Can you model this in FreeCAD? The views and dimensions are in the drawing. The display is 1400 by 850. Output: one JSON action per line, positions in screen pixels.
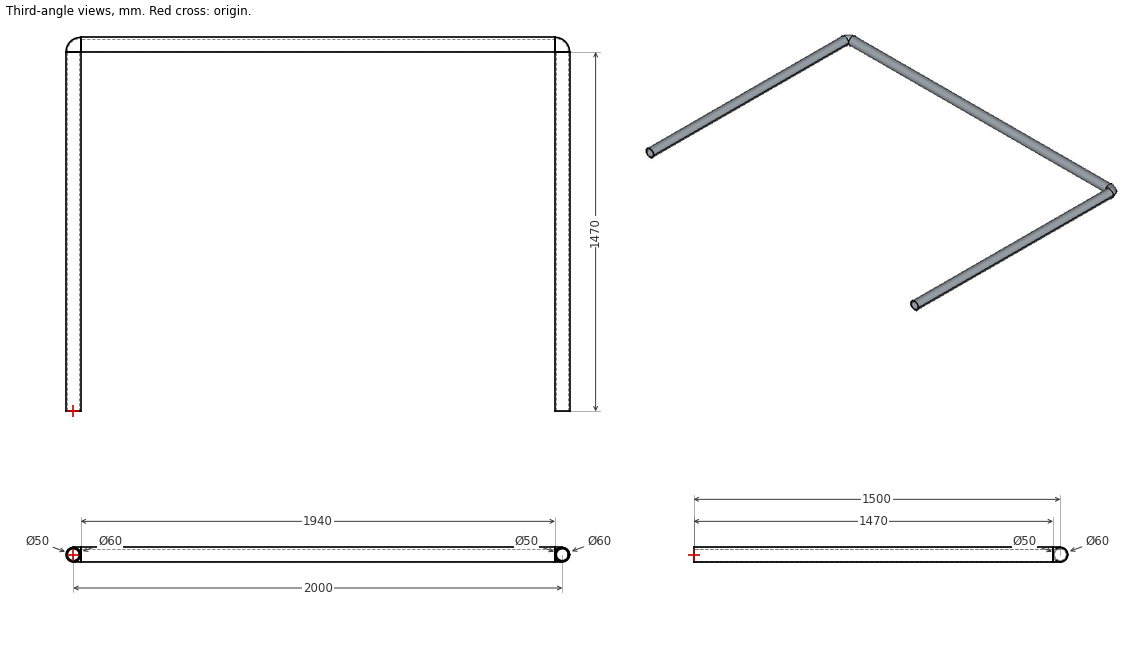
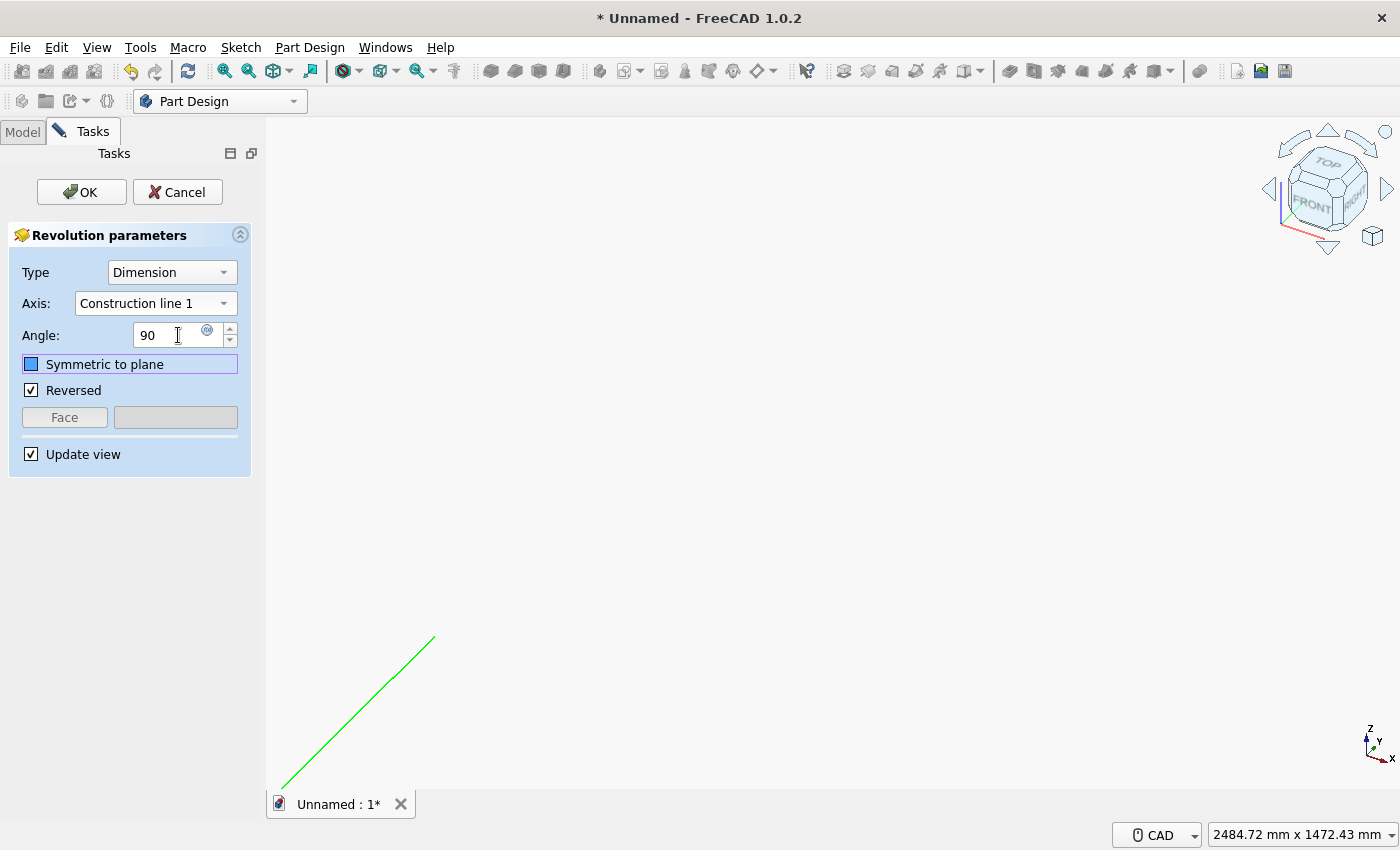
{"action": "left_click", "coordinate": [30, 390]}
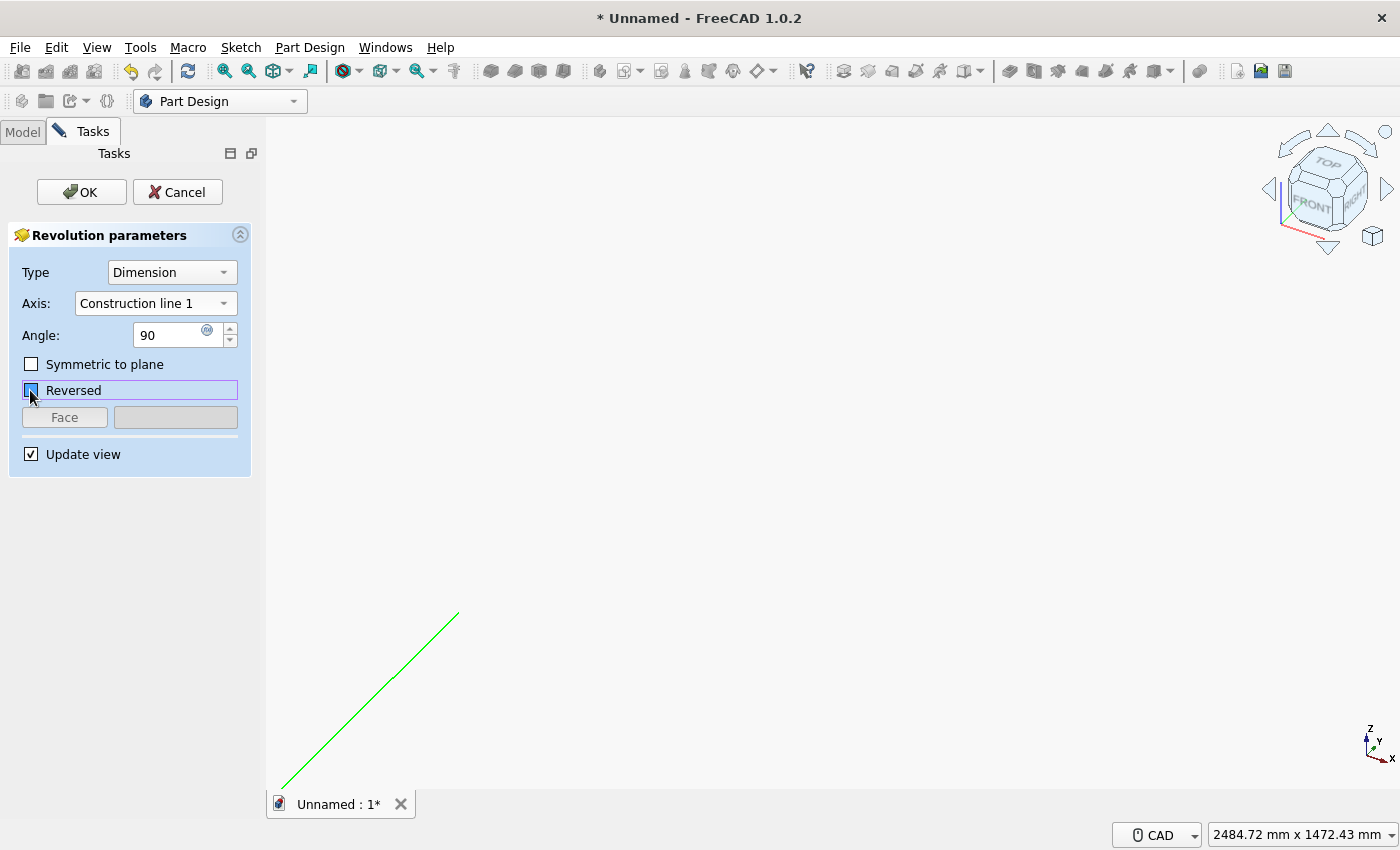
{"action": "left_click", "coordinate": [82, 192]}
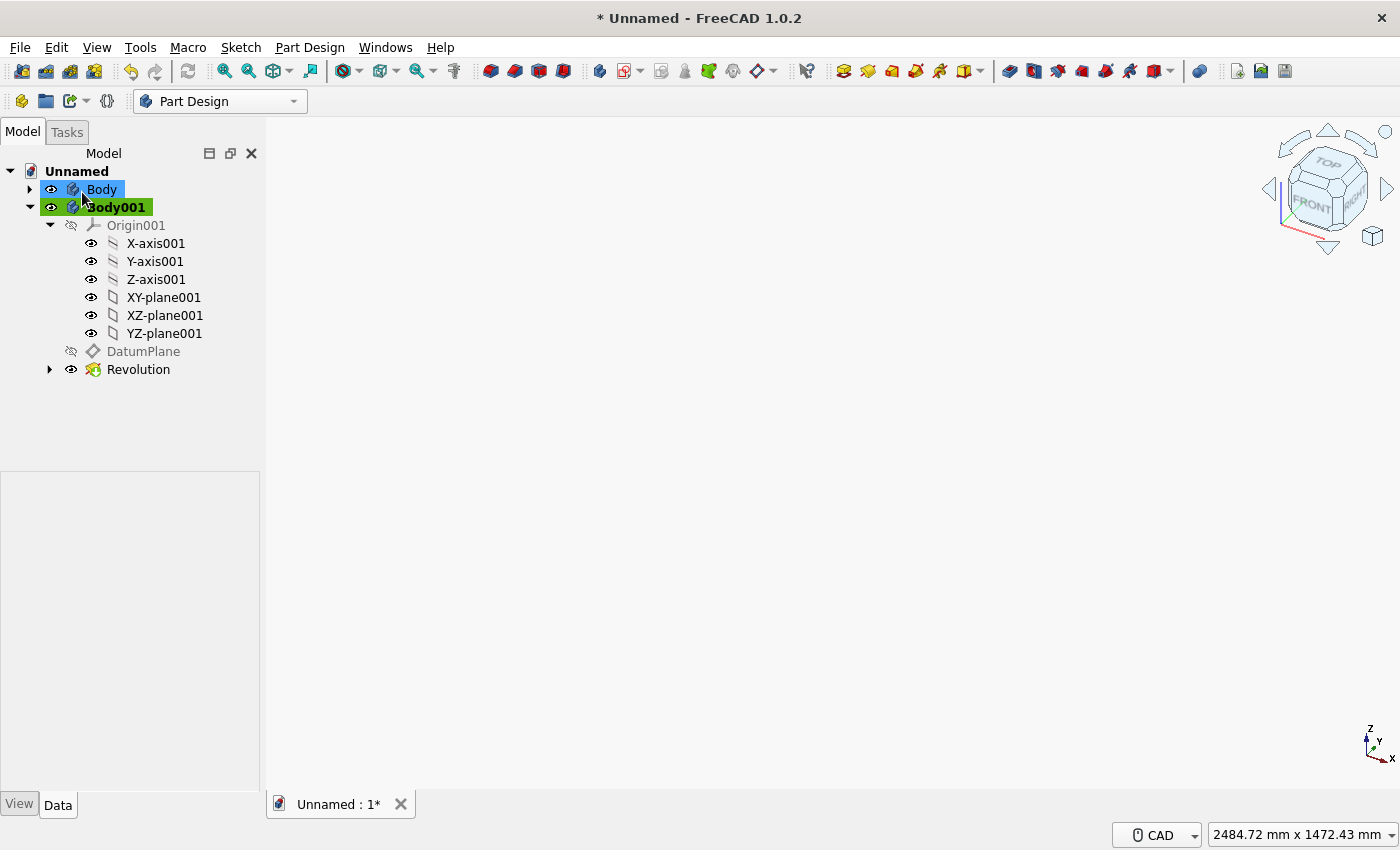
{"action": "left_click", "coordinate": [226, 72]}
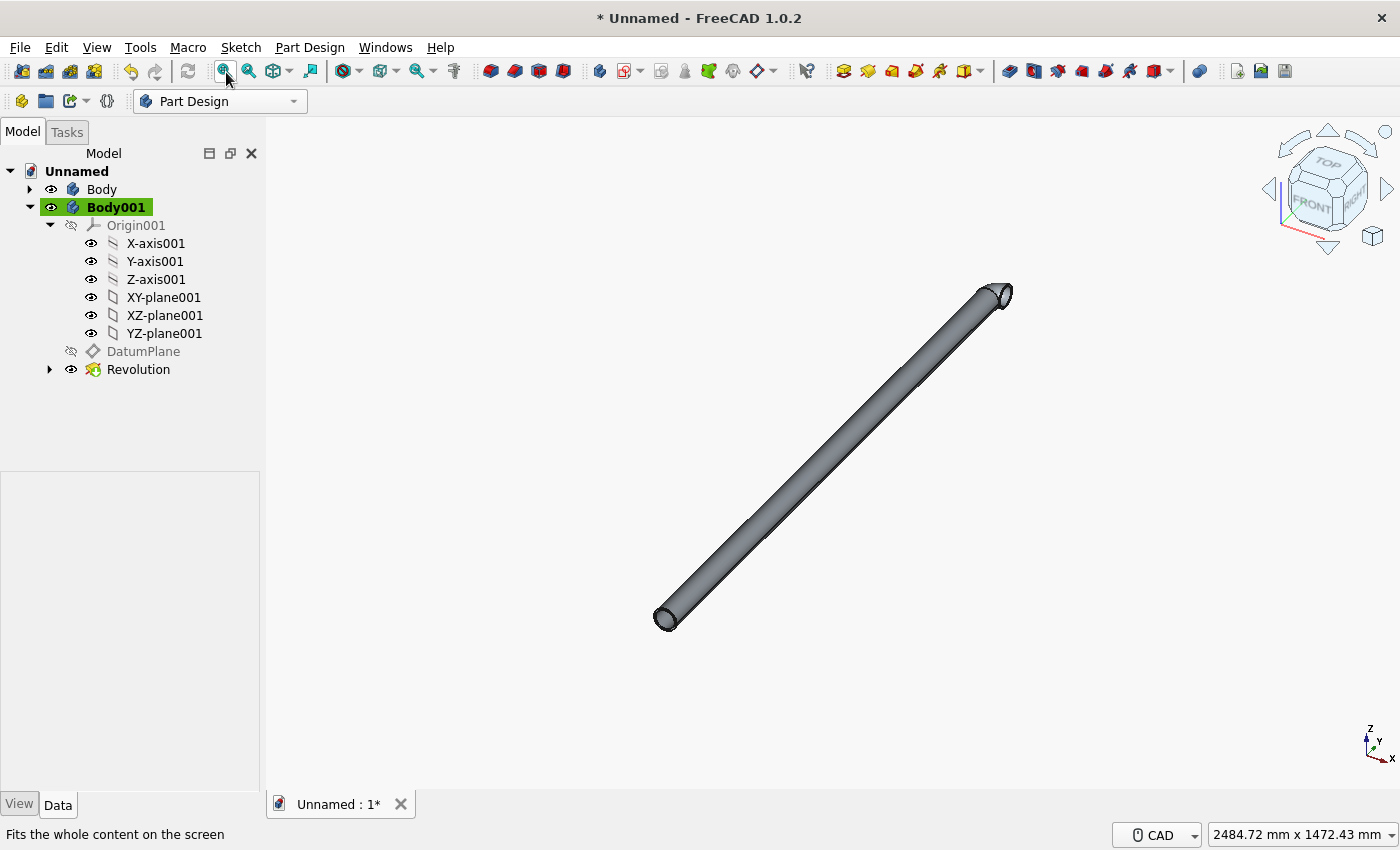
{"action": "left_click", "coordinate": [600, 72]}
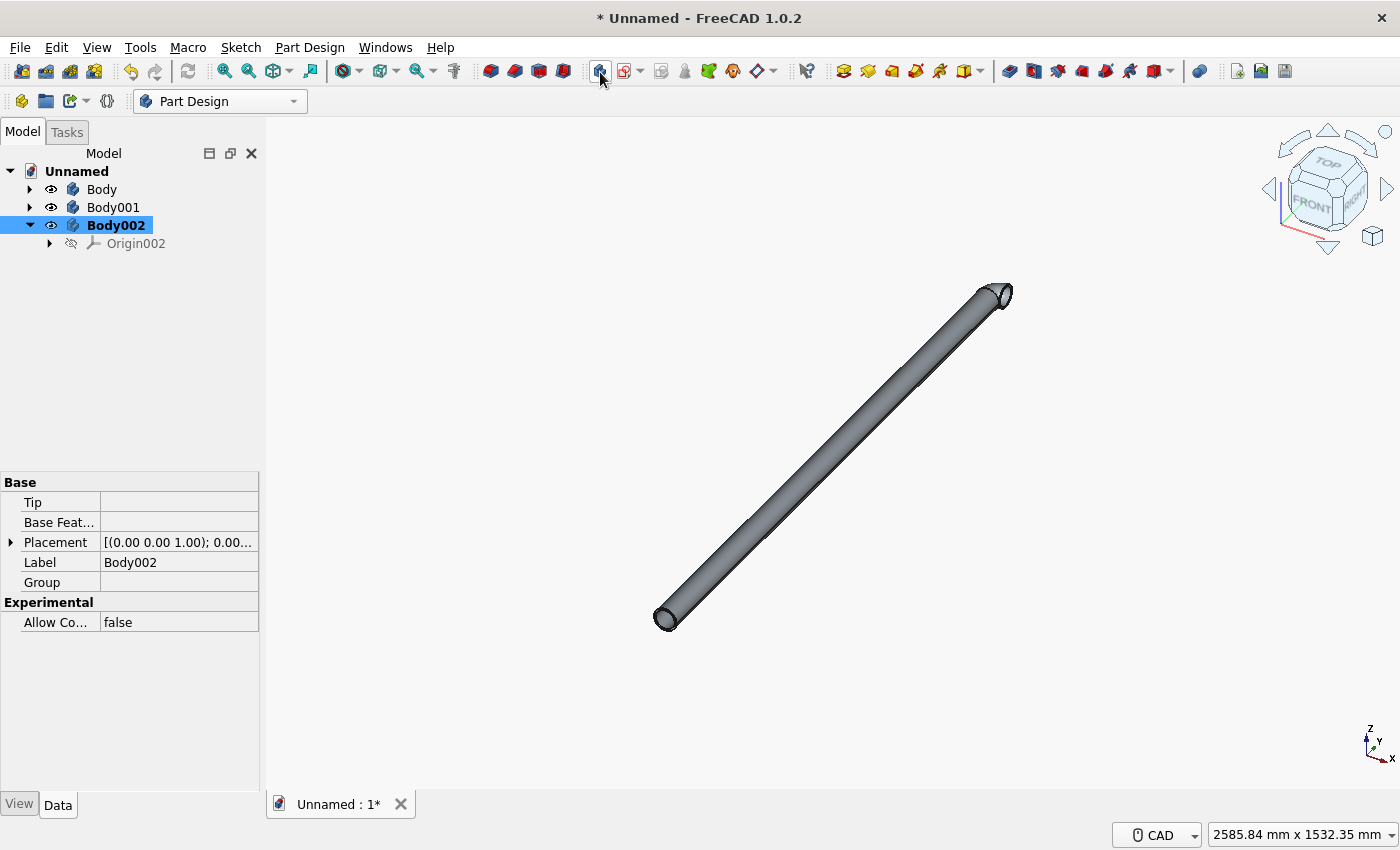
{"action": "left_click", "coordinate": [50, 243]}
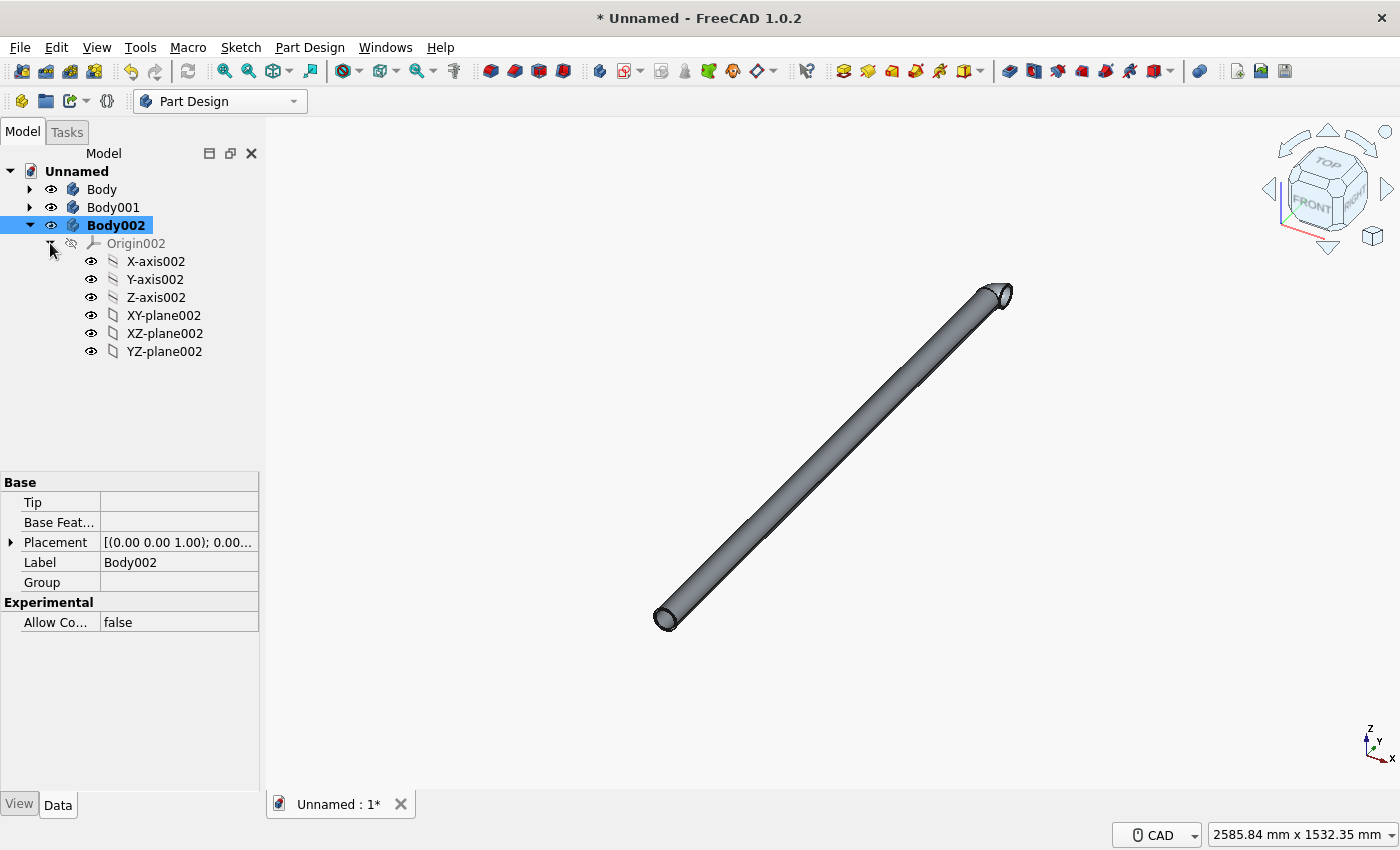
{"action": "left_click", "coordinate": [136, 351]}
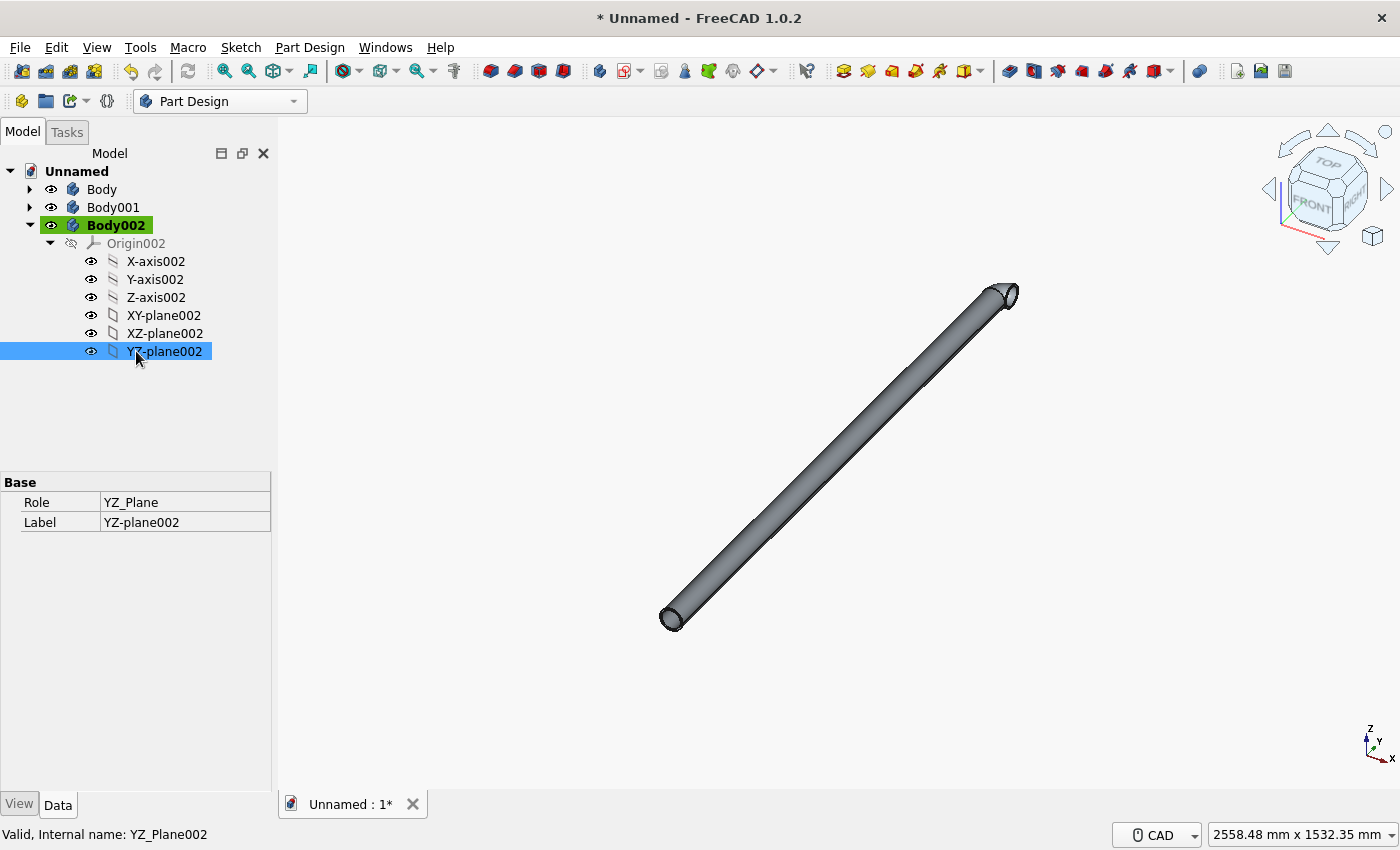
{"action": "left_click", "coordinate": [758, 72]}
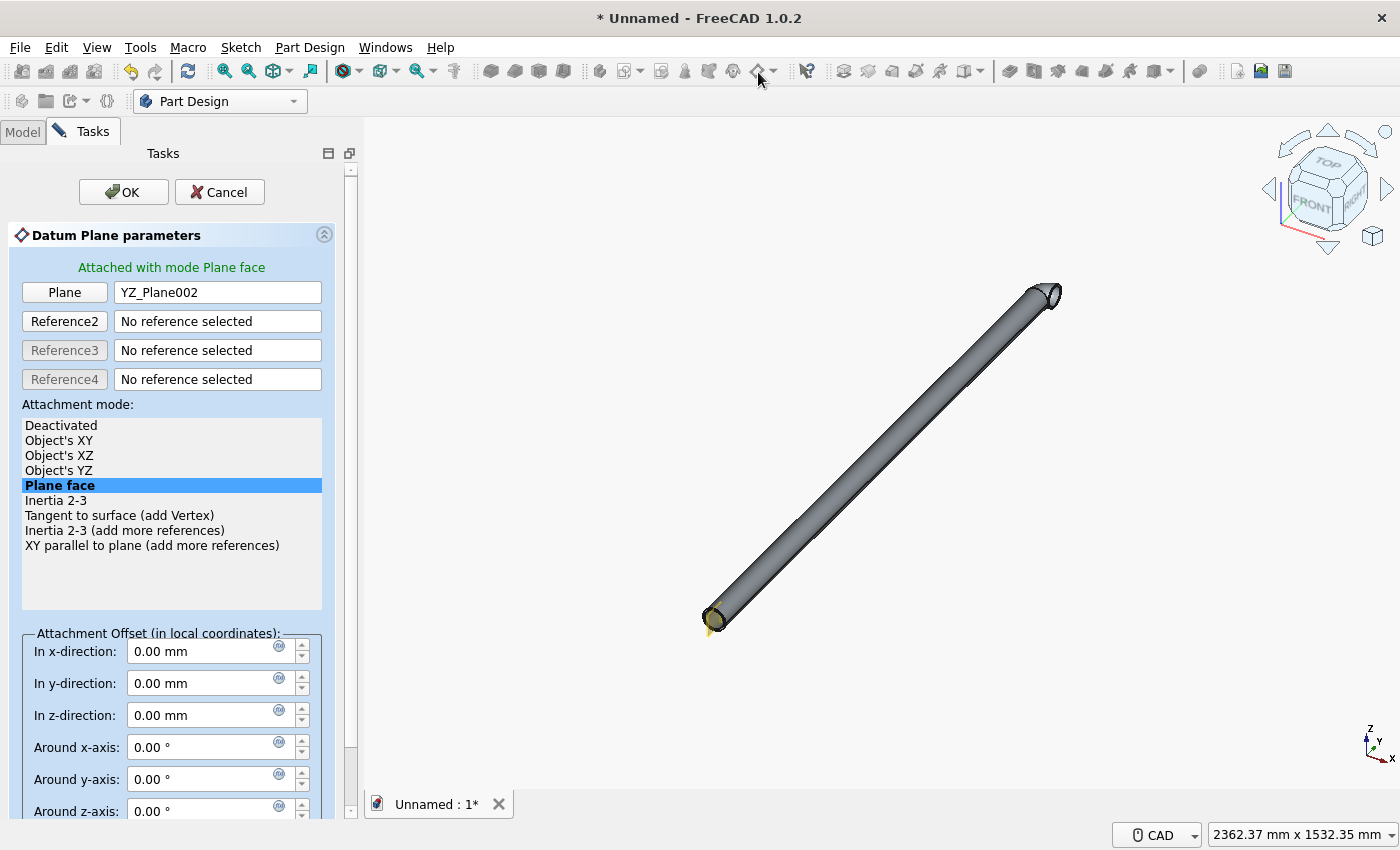
{"action": "triple_click", "coordinate": [210, 715]}